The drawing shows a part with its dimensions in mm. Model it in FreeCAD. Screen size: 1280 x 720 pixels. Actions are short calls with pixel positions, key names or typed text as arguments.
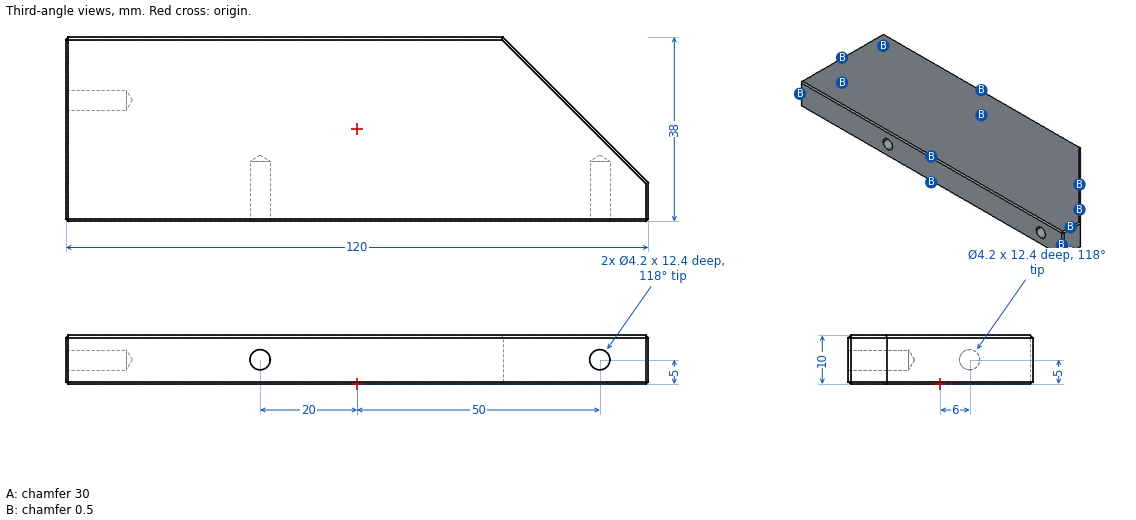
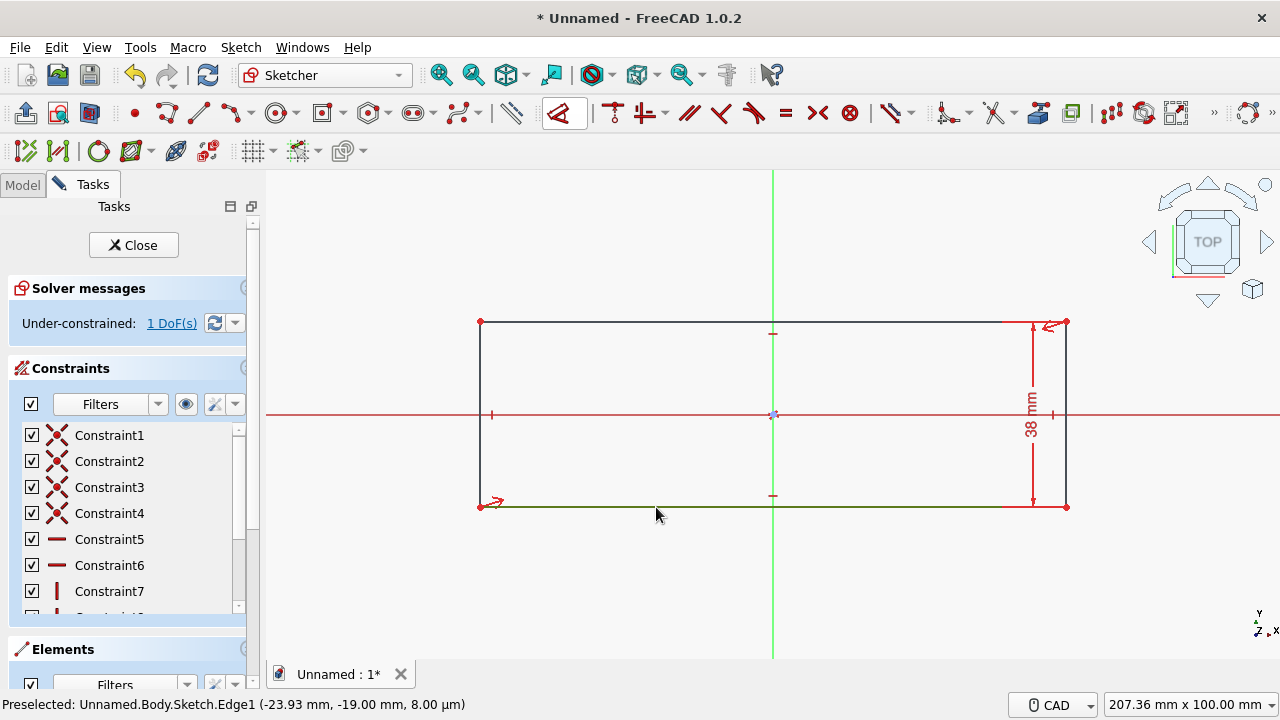
click(582, 114)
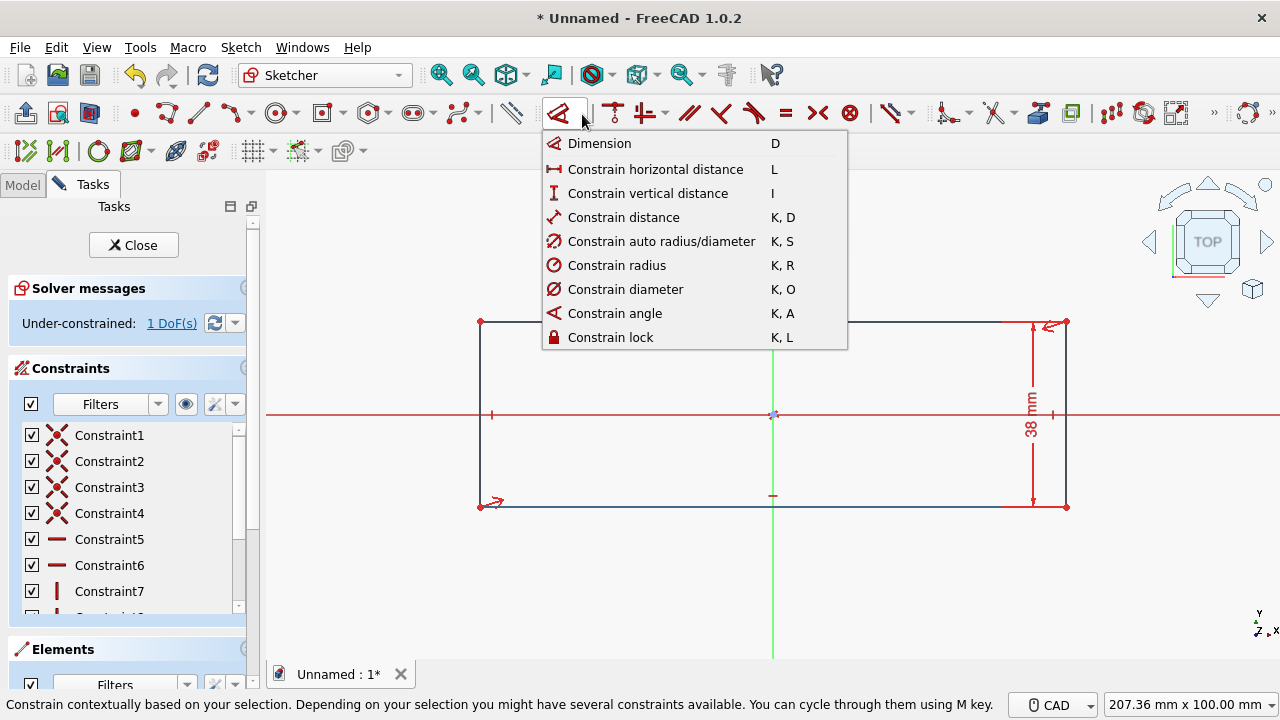
click(695, 169)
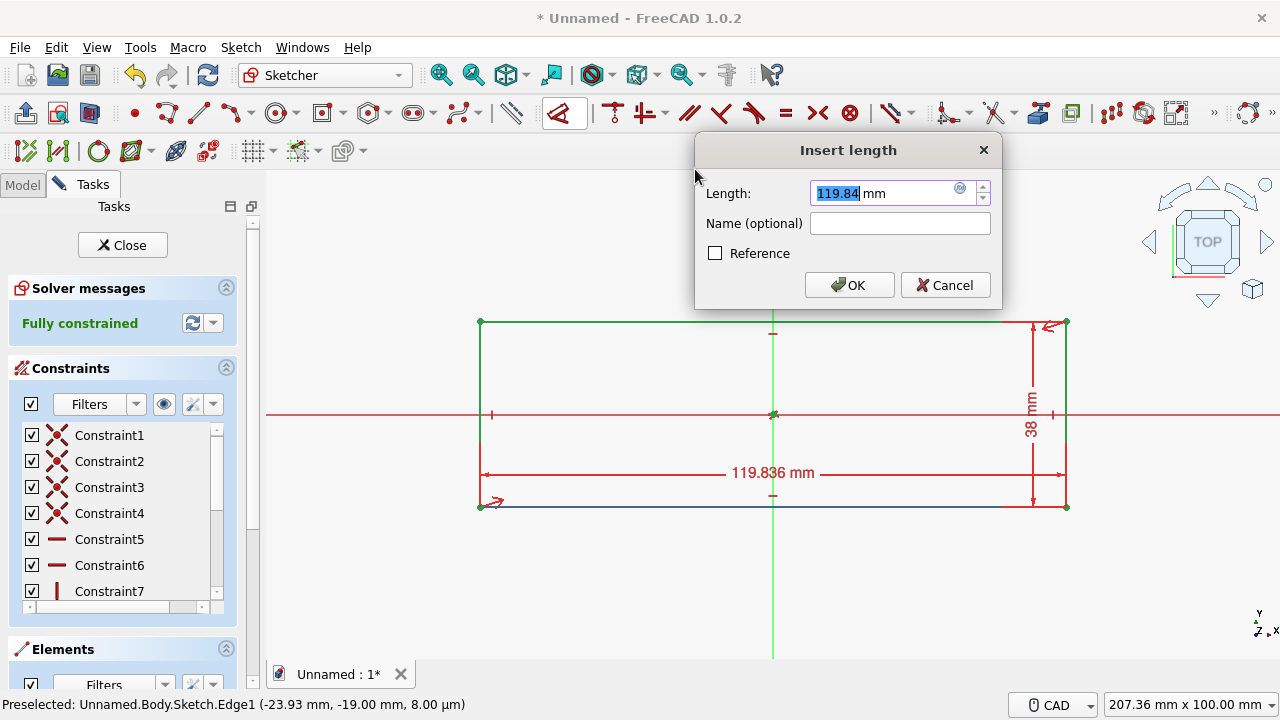
text(120)
key(Return)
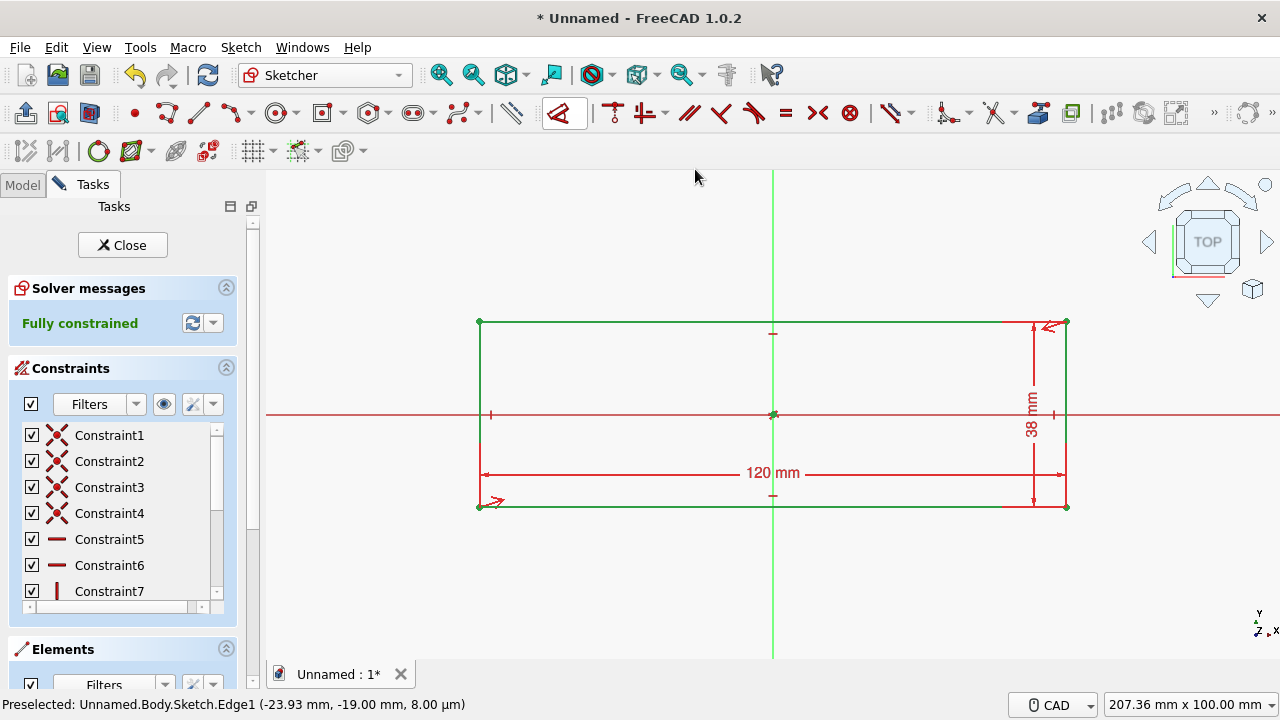
click(123, 245)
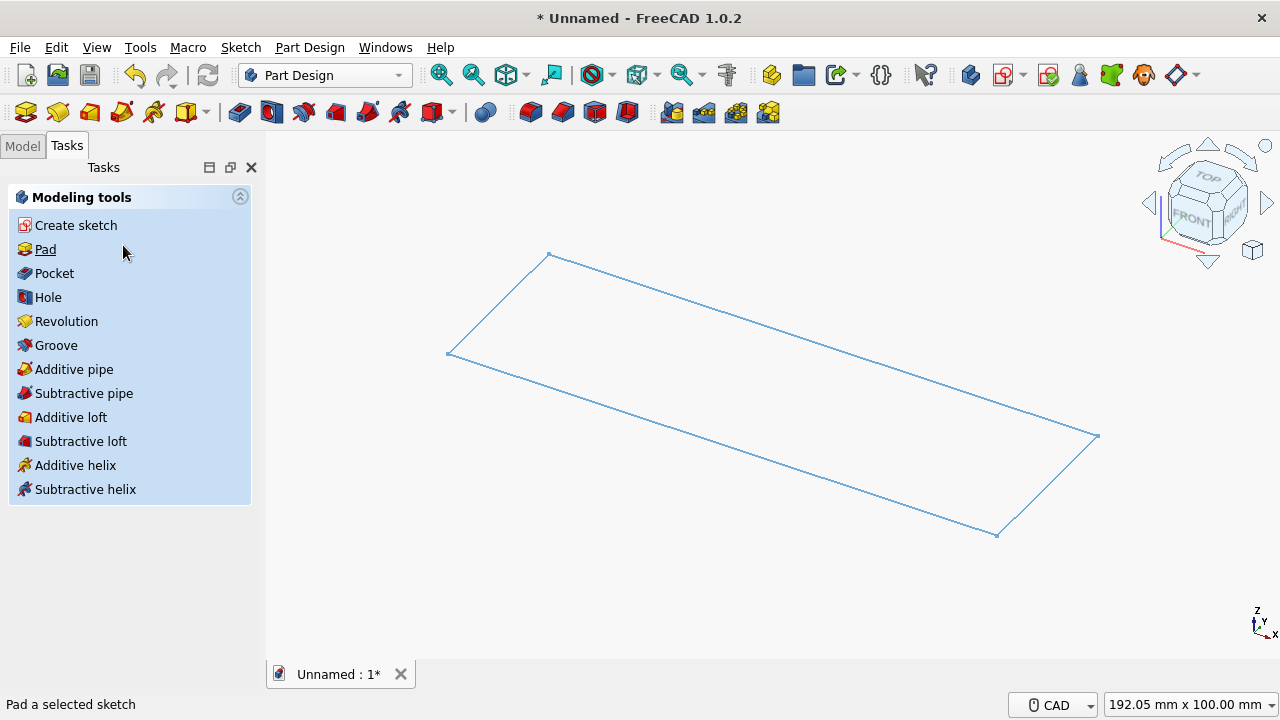
click(26, 112)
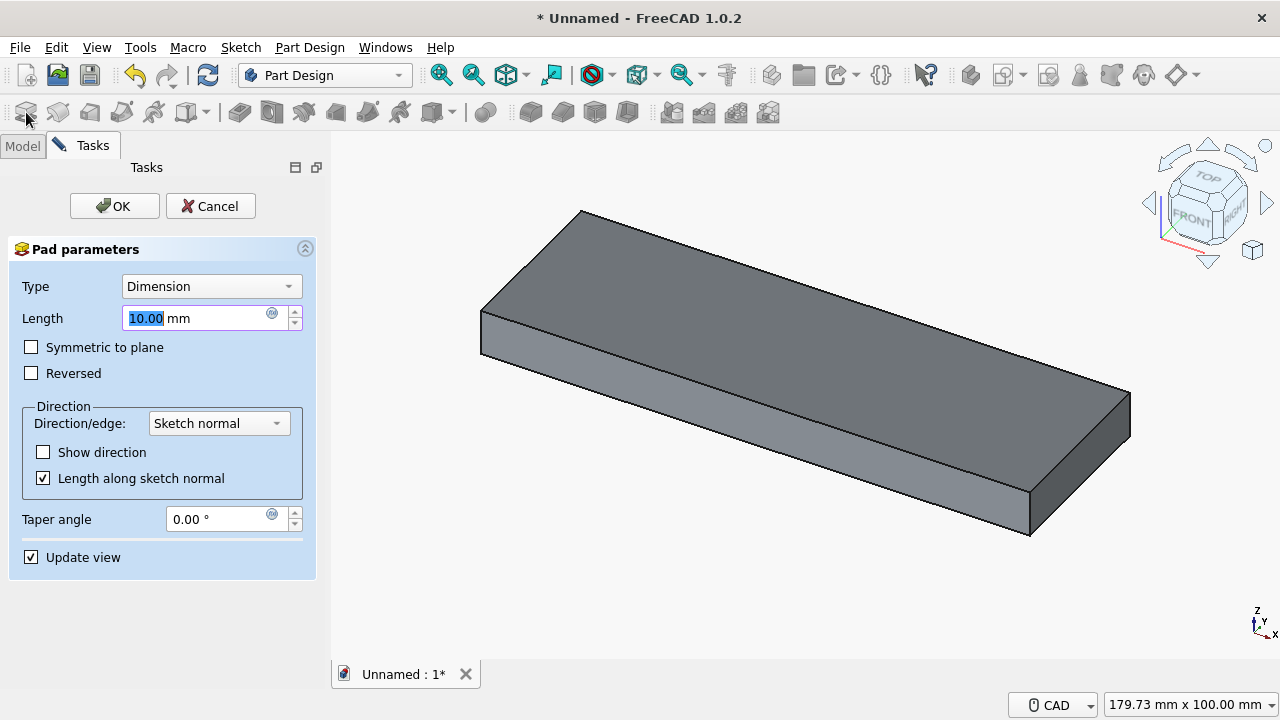
text(10)
key(Tab)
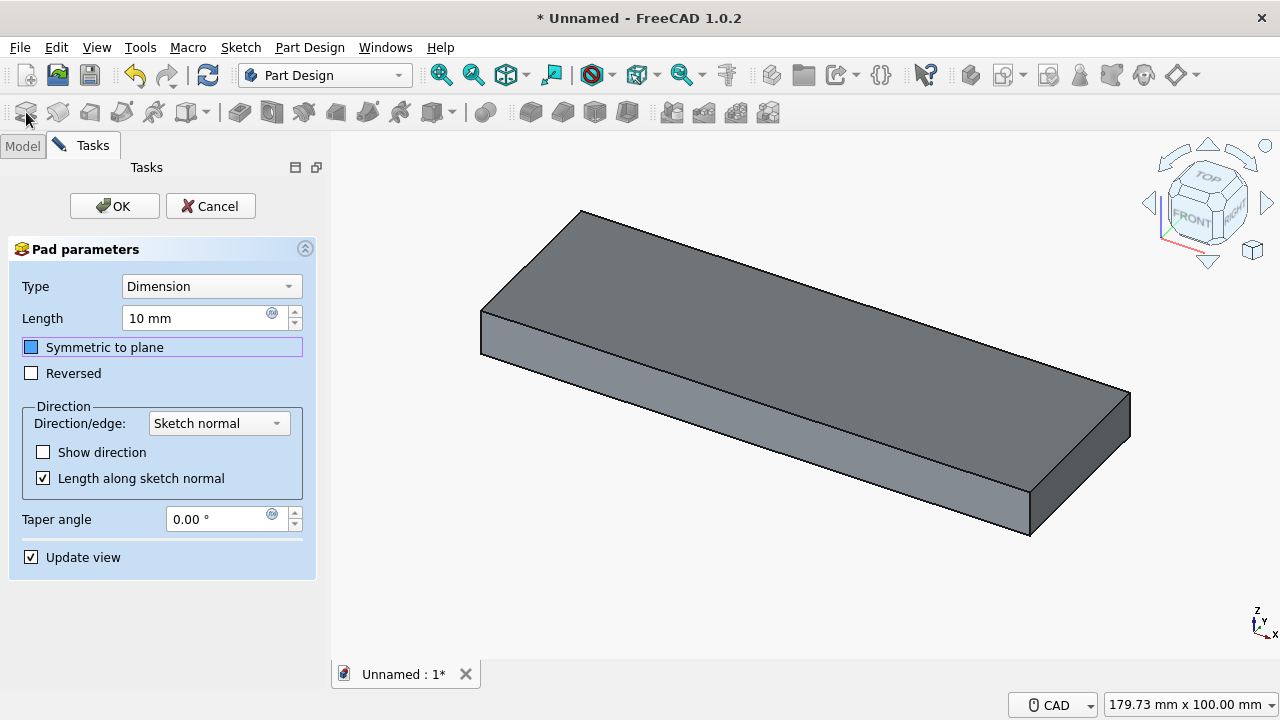
click(115, 206)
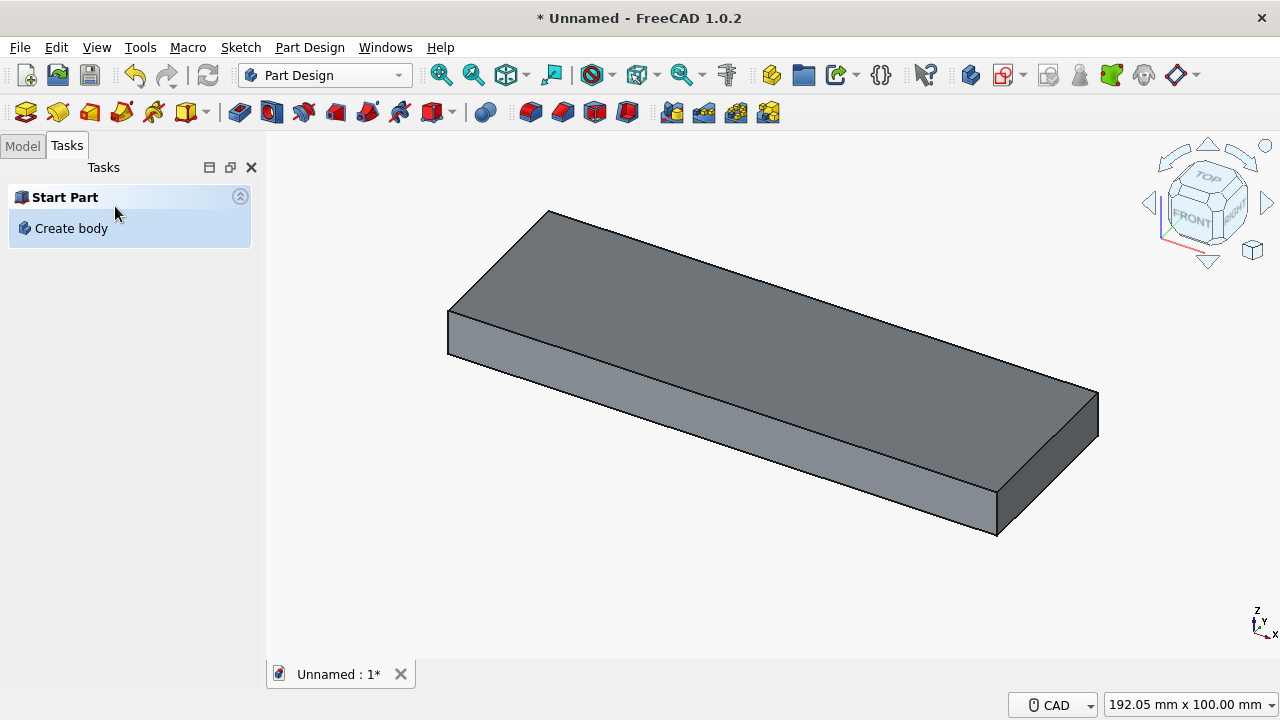
key(0)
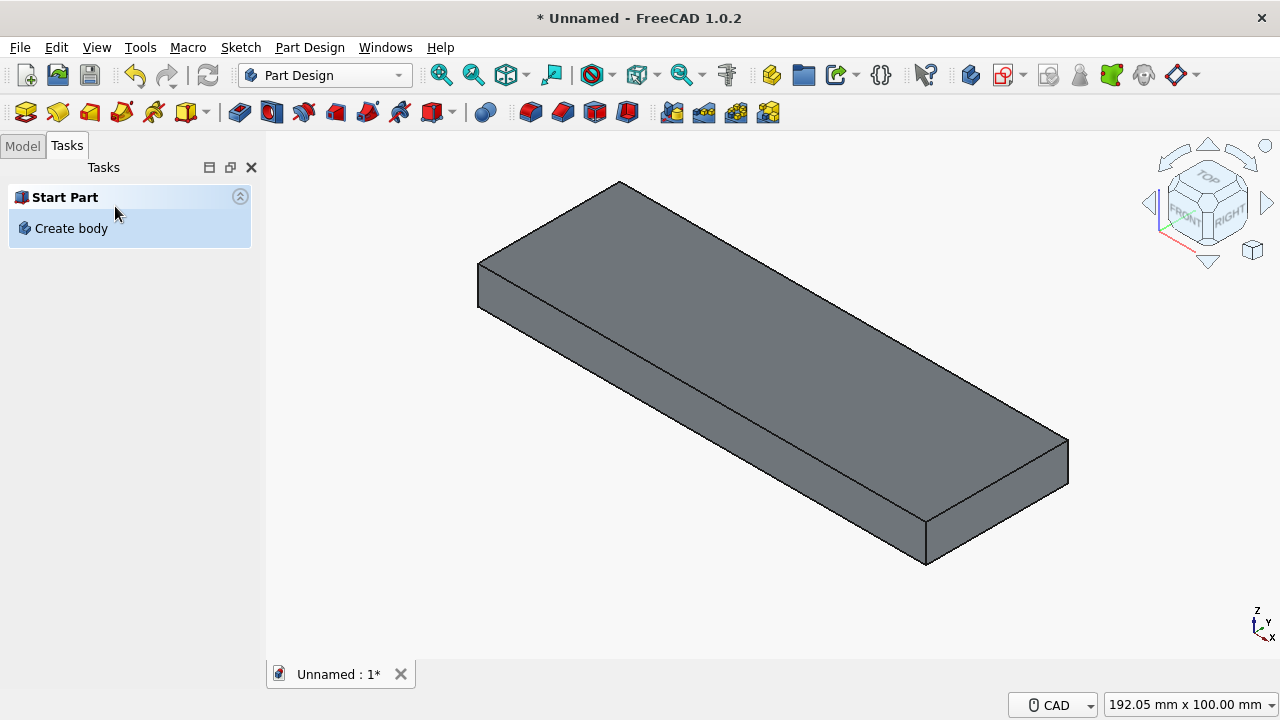
key(2)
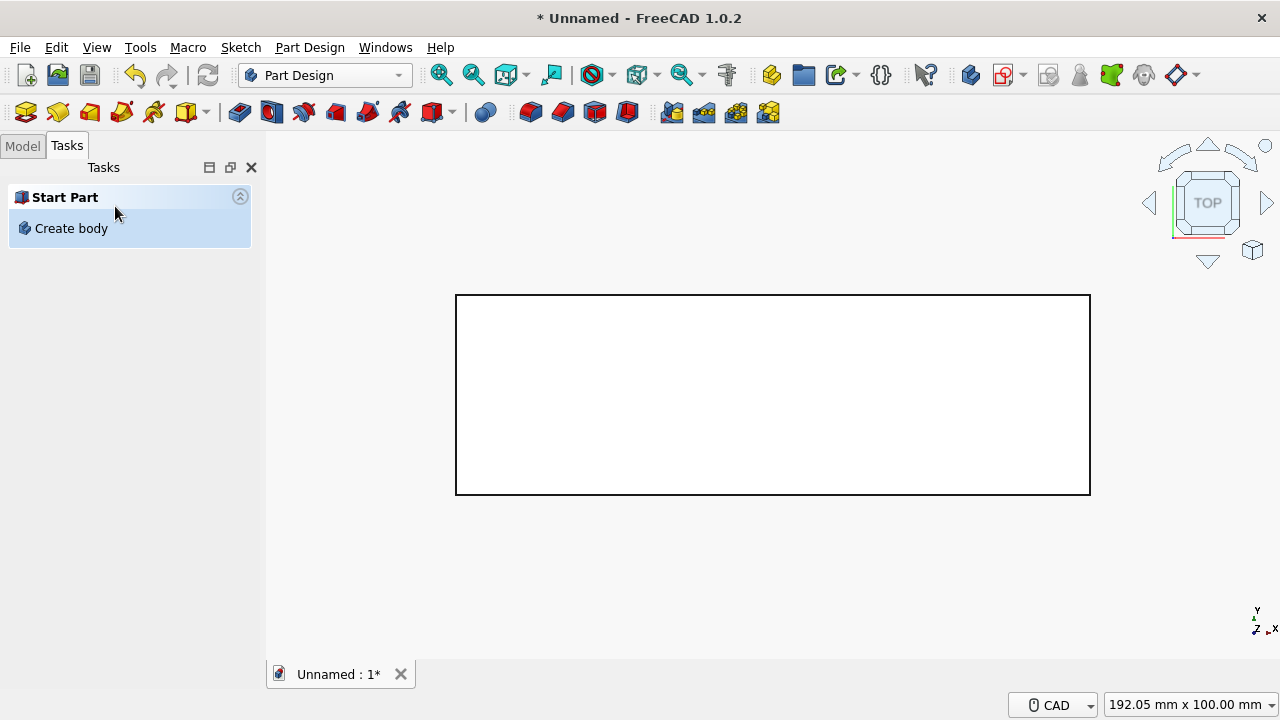
key(1)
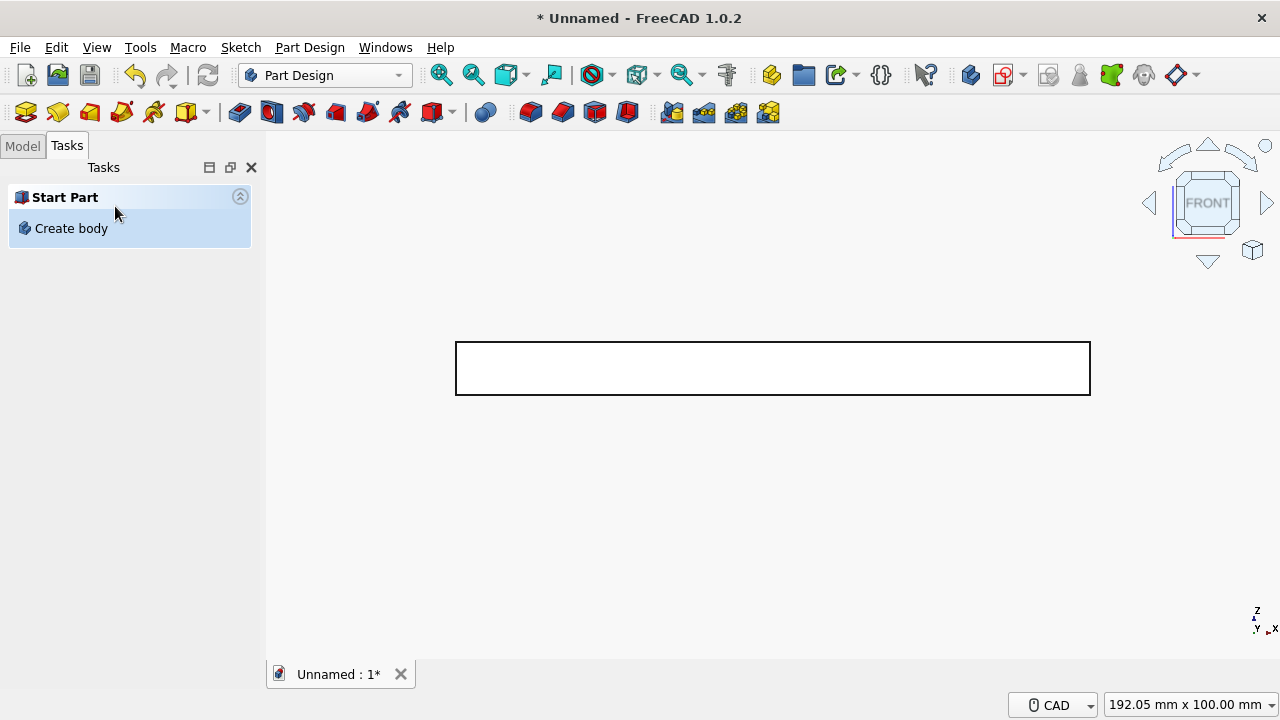
key(3)